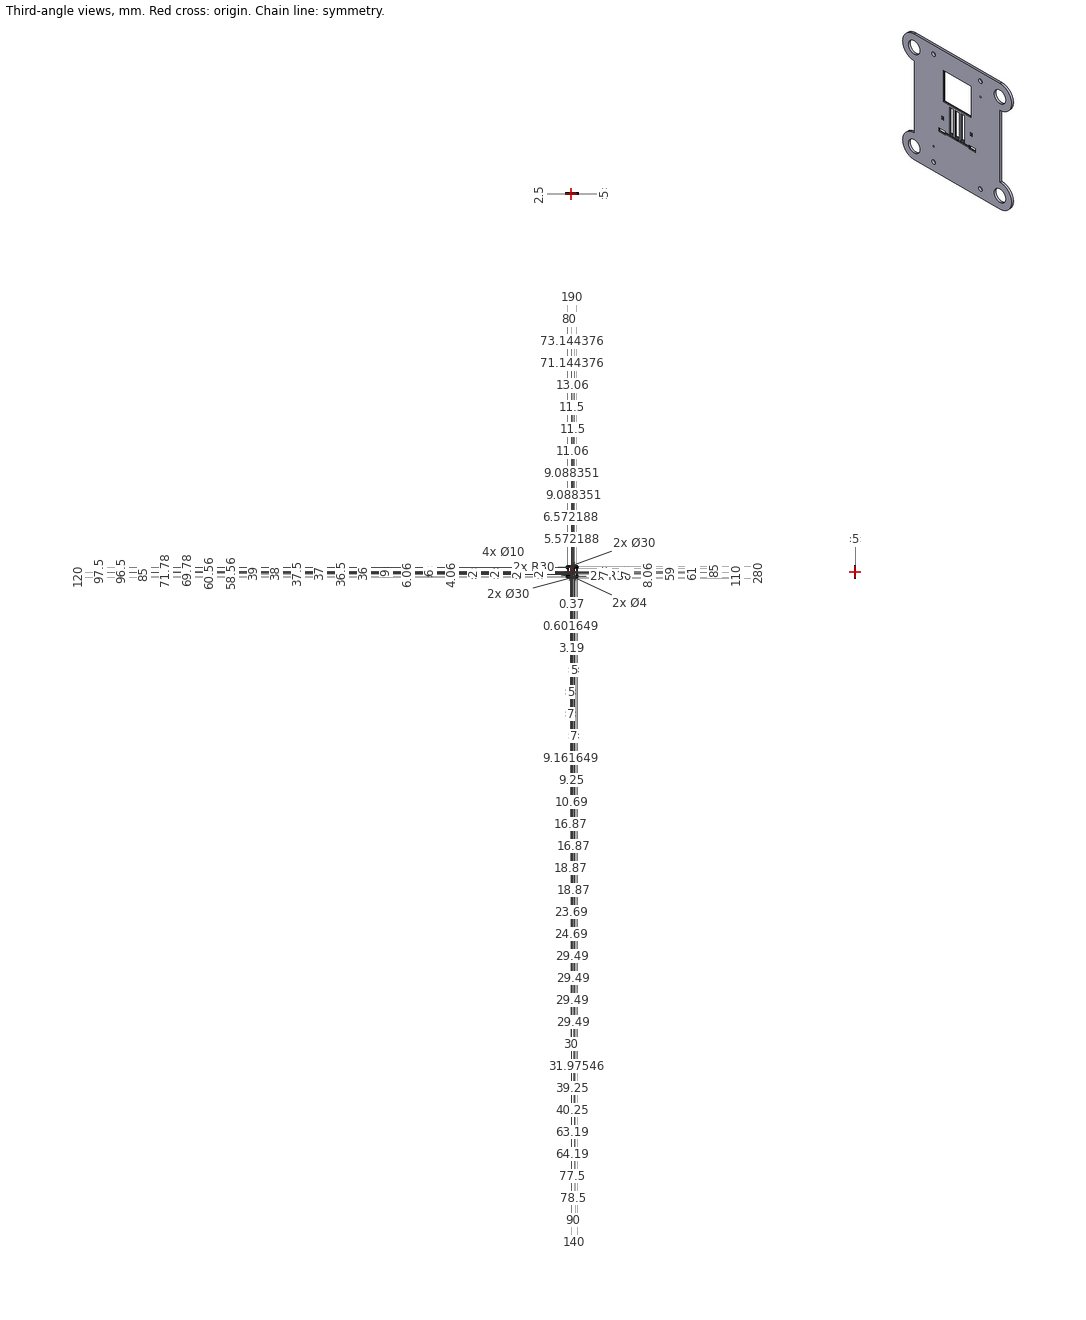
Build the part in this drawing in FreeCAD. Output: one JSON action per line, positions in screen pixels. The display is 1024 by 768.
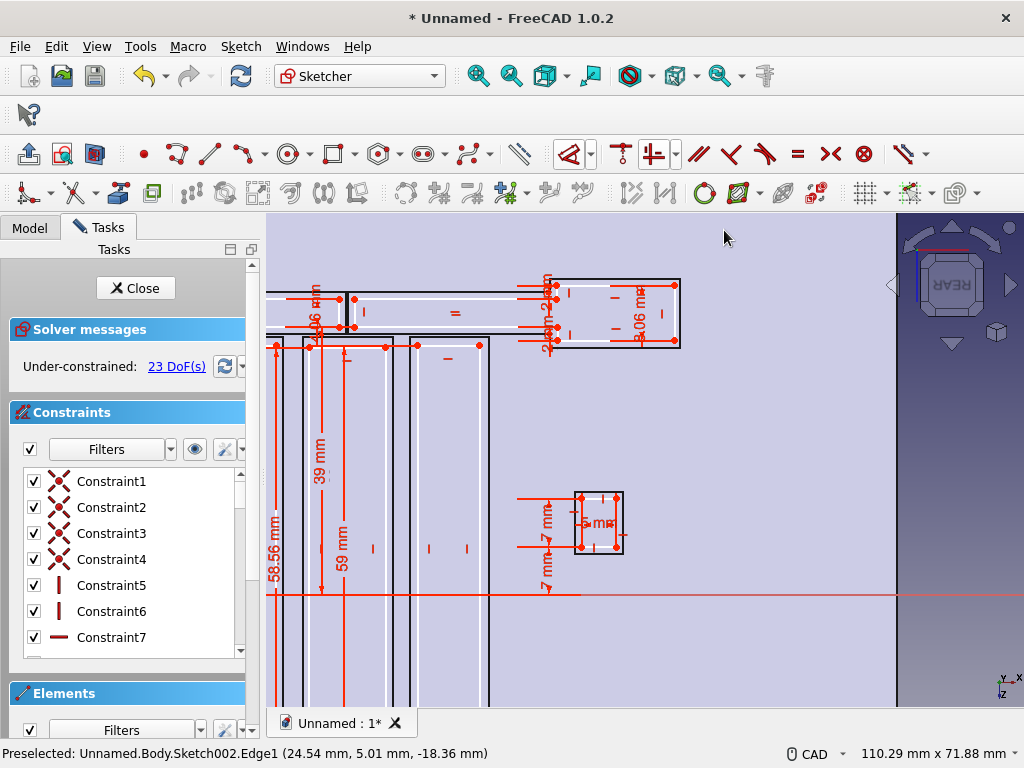
{"action": "scroll", "coordinate": [675, 326], "scroll_direction": "down", "scroll_amount": 6}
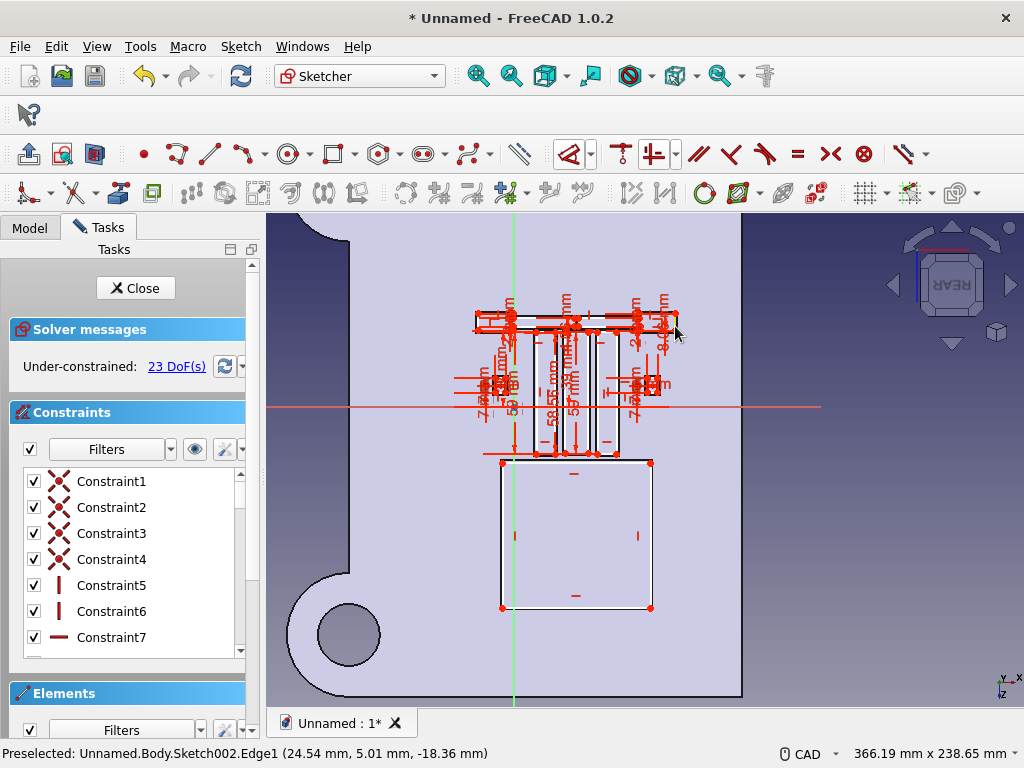
{"action": "scroll", "coordinate": [572, 454], "scroll_direction": "up", "scroll_amount": 4}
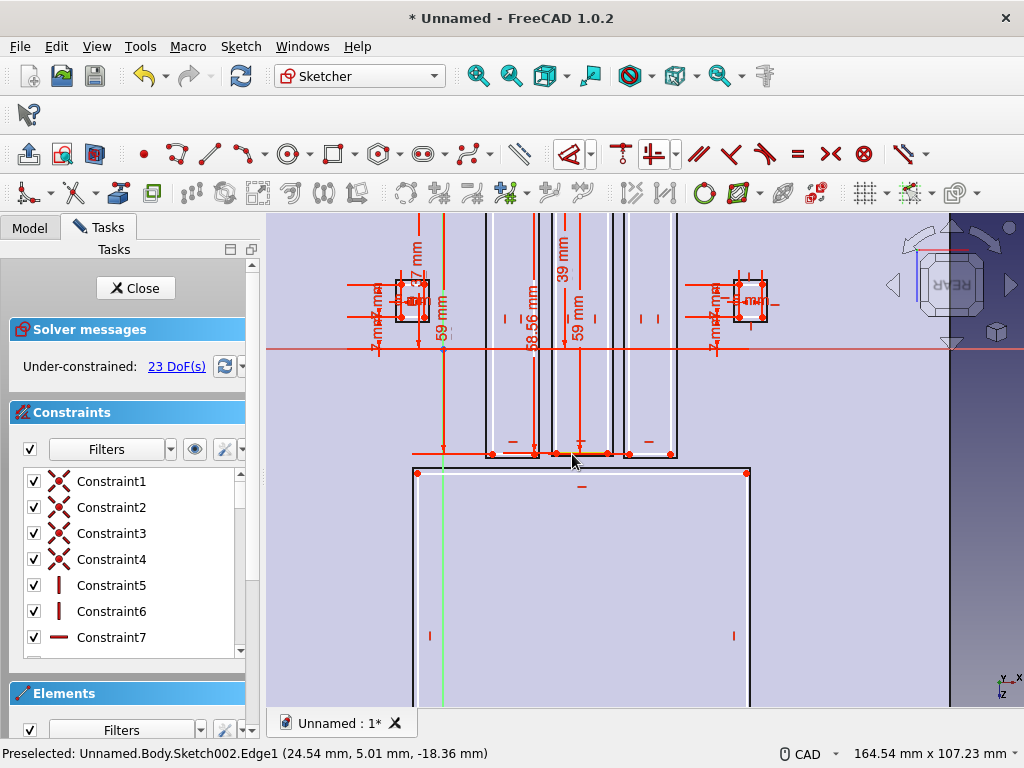
{"action": "left_click", "coordinate": [572, 453]}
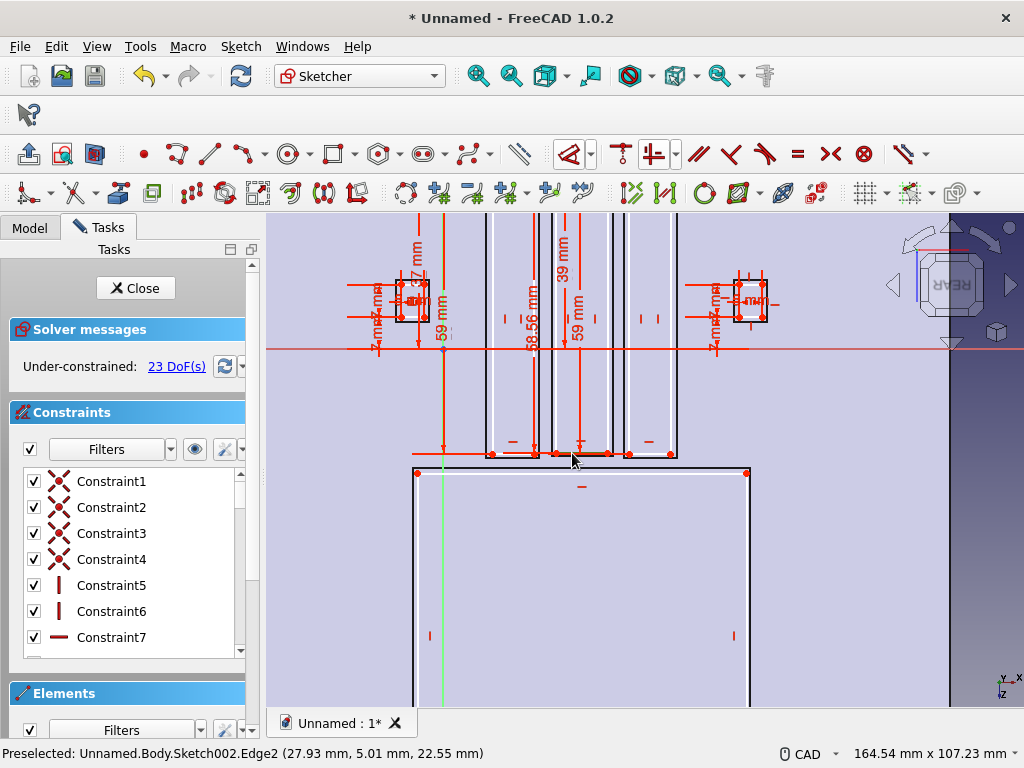
{"action": "left_click", "coordinate": [590, 154]}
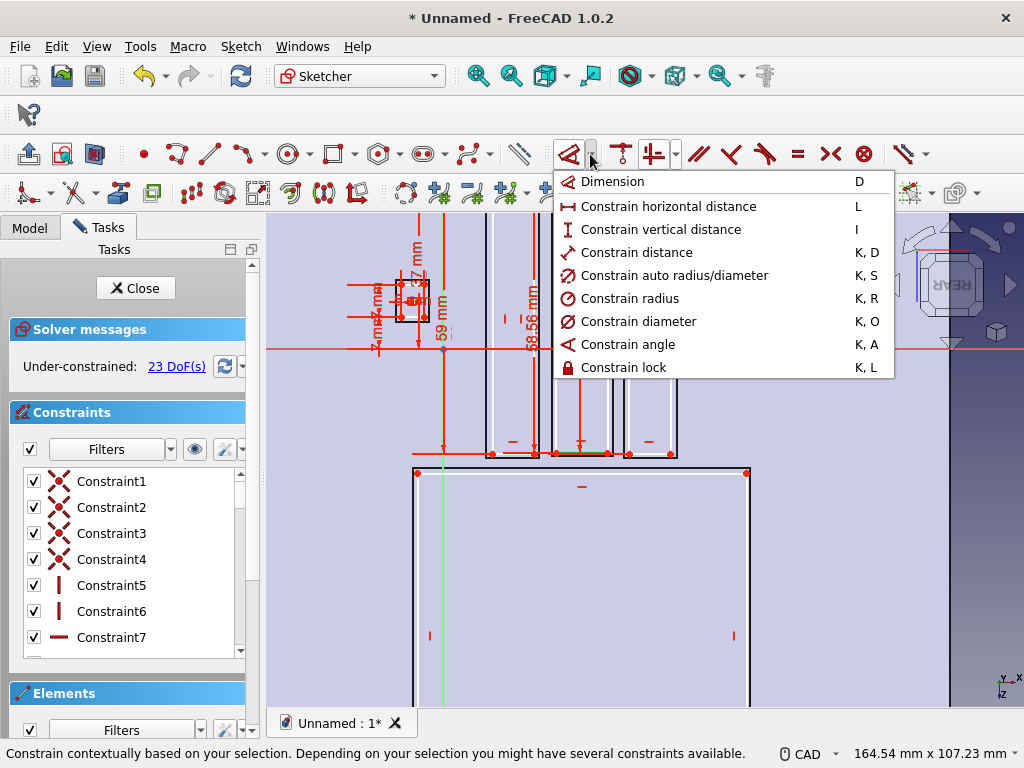
{"action": "left_click", "coordinate": [724, 206]}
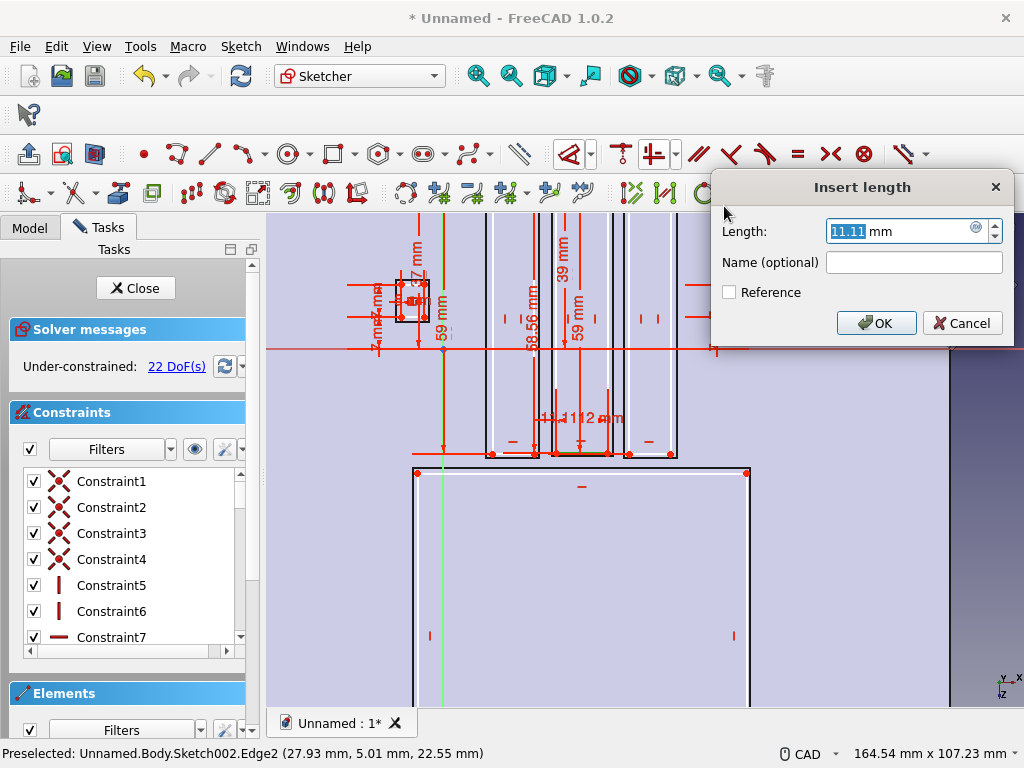
{"action": "type", "text": "11.06"}
{"action": "key", "text": "Return"}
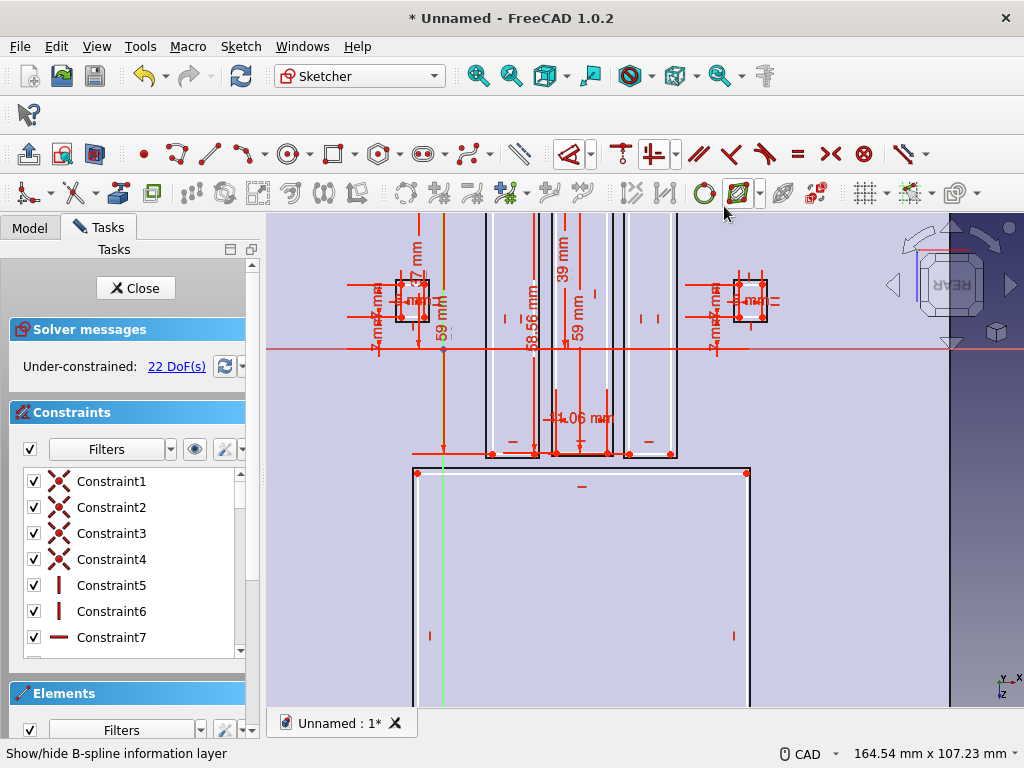
{"action": "scroll", "coordinate": [572, 454], "scroll_direction": "down", "scroll_amount": 4}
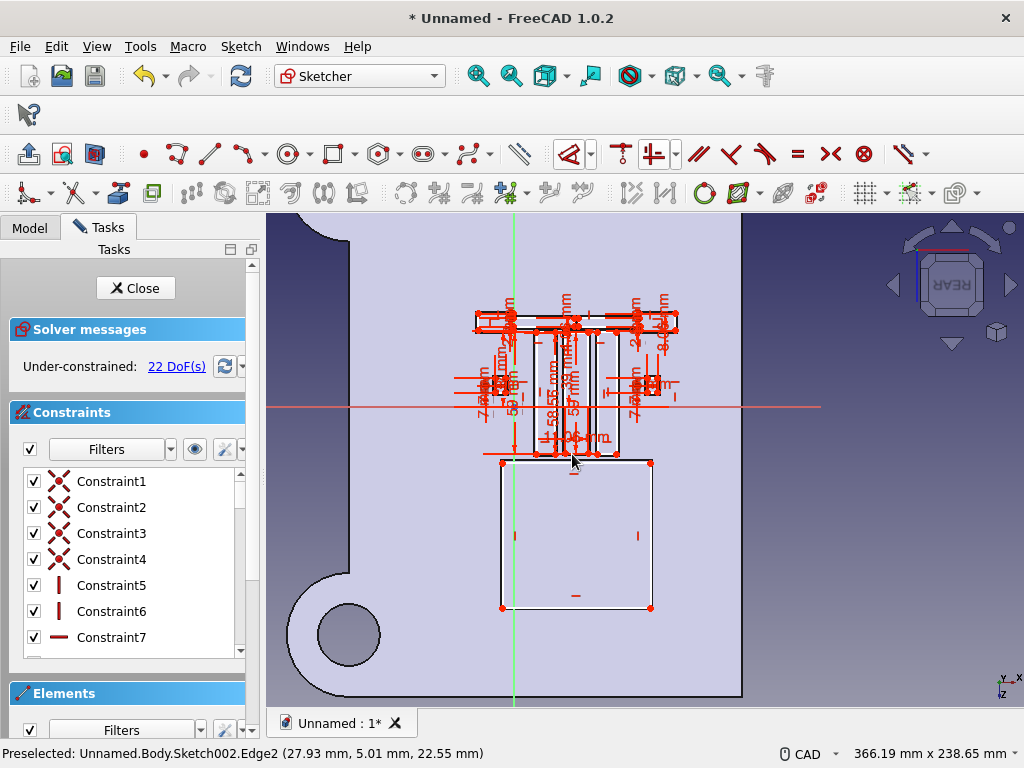
{"action": "scroll", "coordinate": [532, 327], "scroll_direction": "up", "scroll_amount": 3}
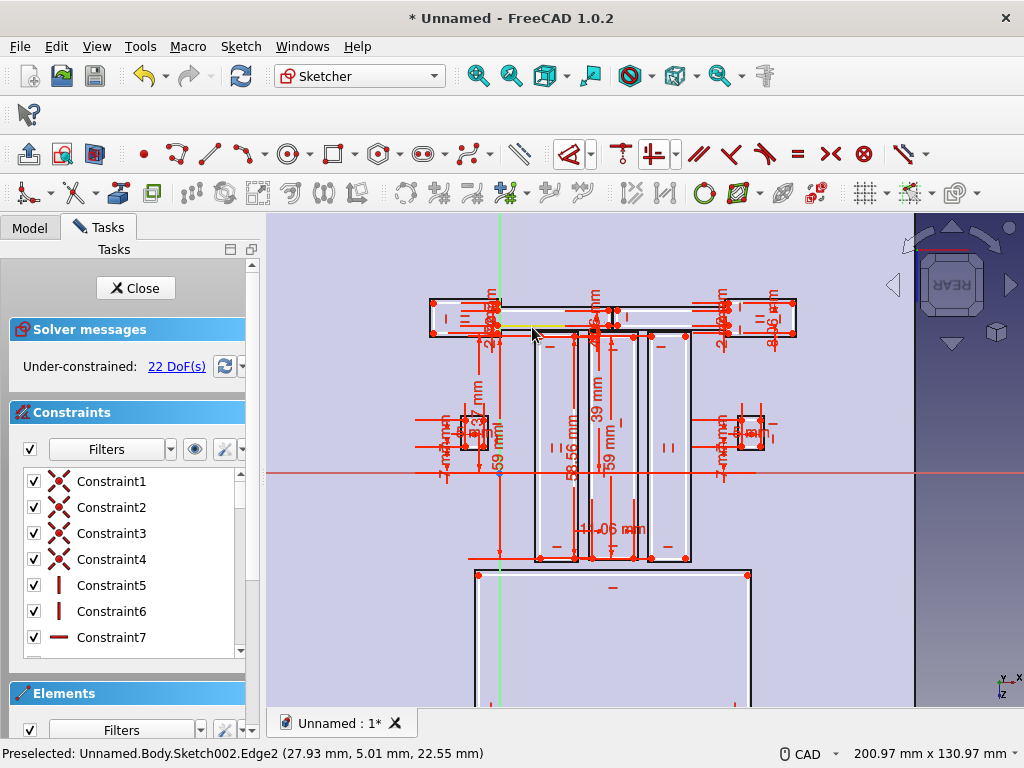
{"action": "left_click", "coordinate": [531, 326]}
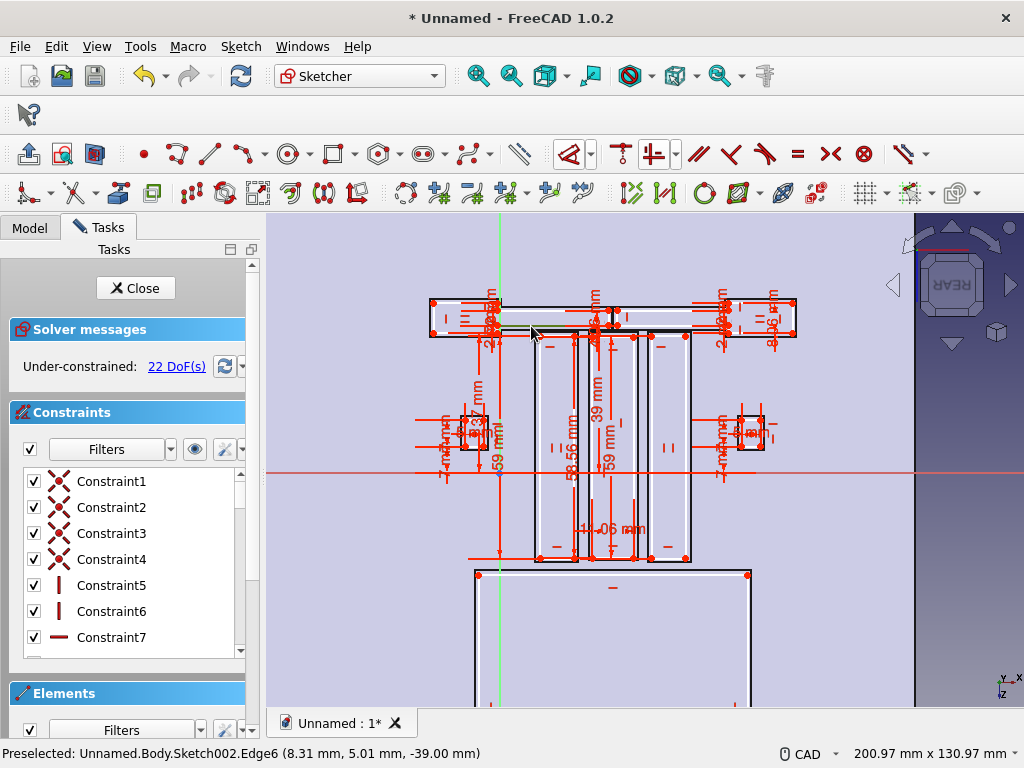
{"action": "left_click", "coordinate": [590, 154]}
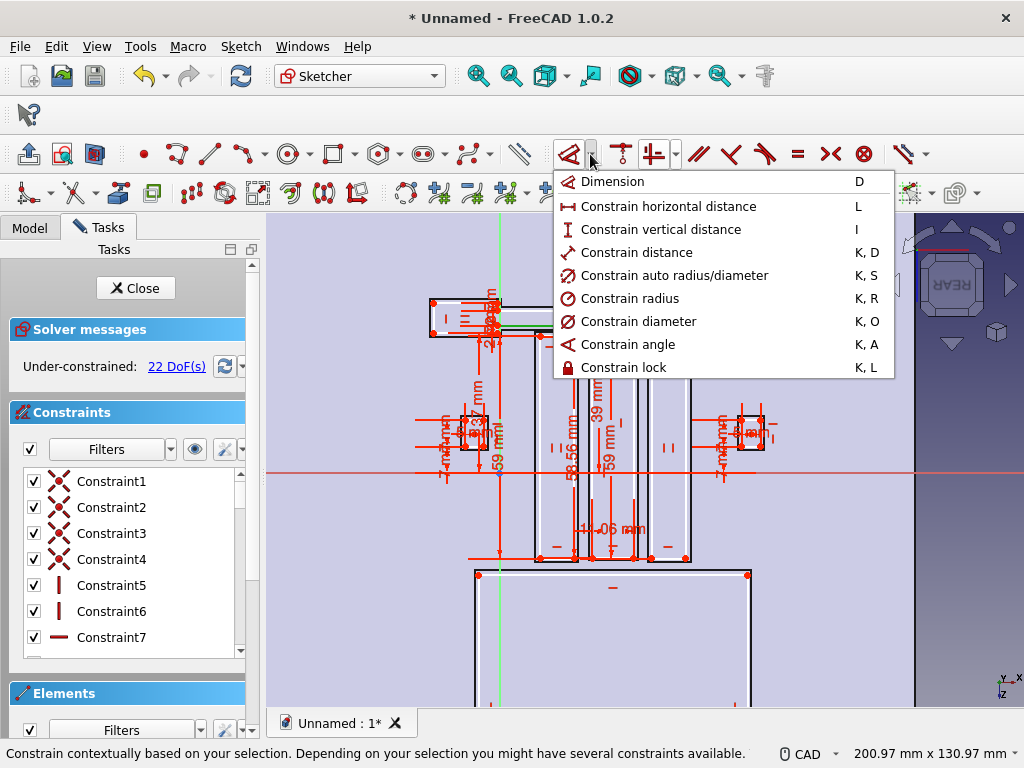
{"action": "left_click", "coordinate": [724, 206]}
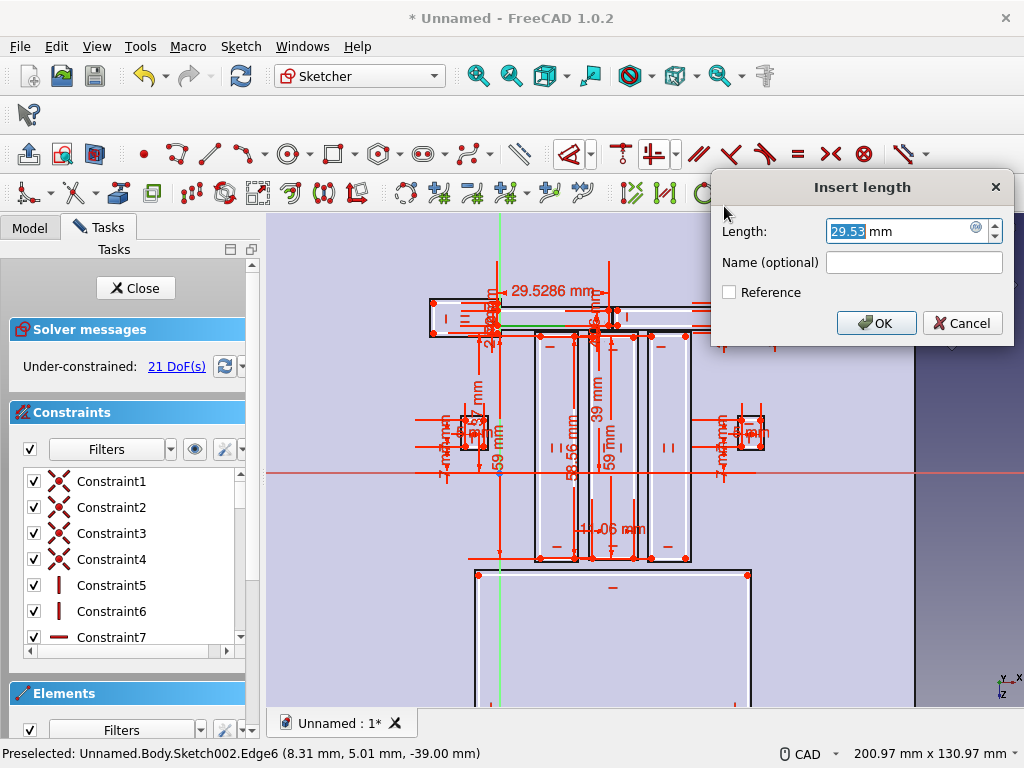
{"action": "type", "text": "29.49"}
{"action": "key", "text": "Return"}